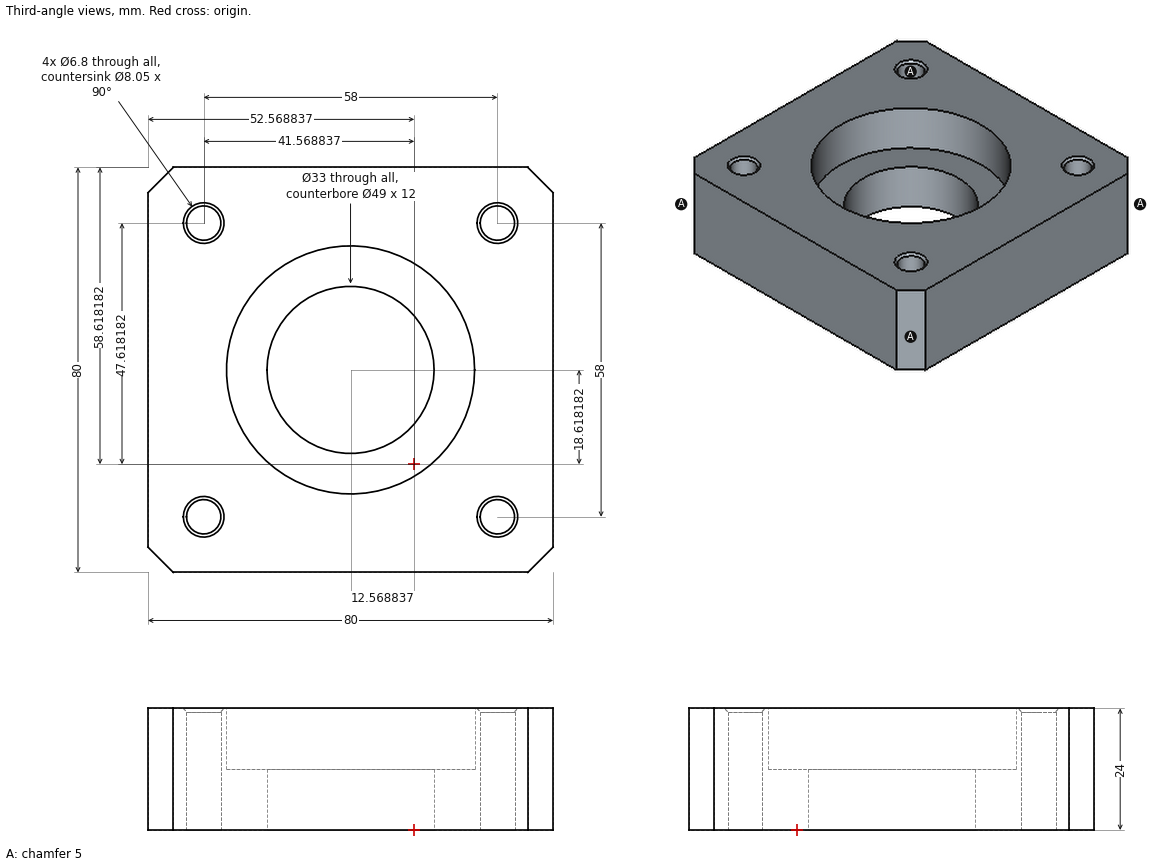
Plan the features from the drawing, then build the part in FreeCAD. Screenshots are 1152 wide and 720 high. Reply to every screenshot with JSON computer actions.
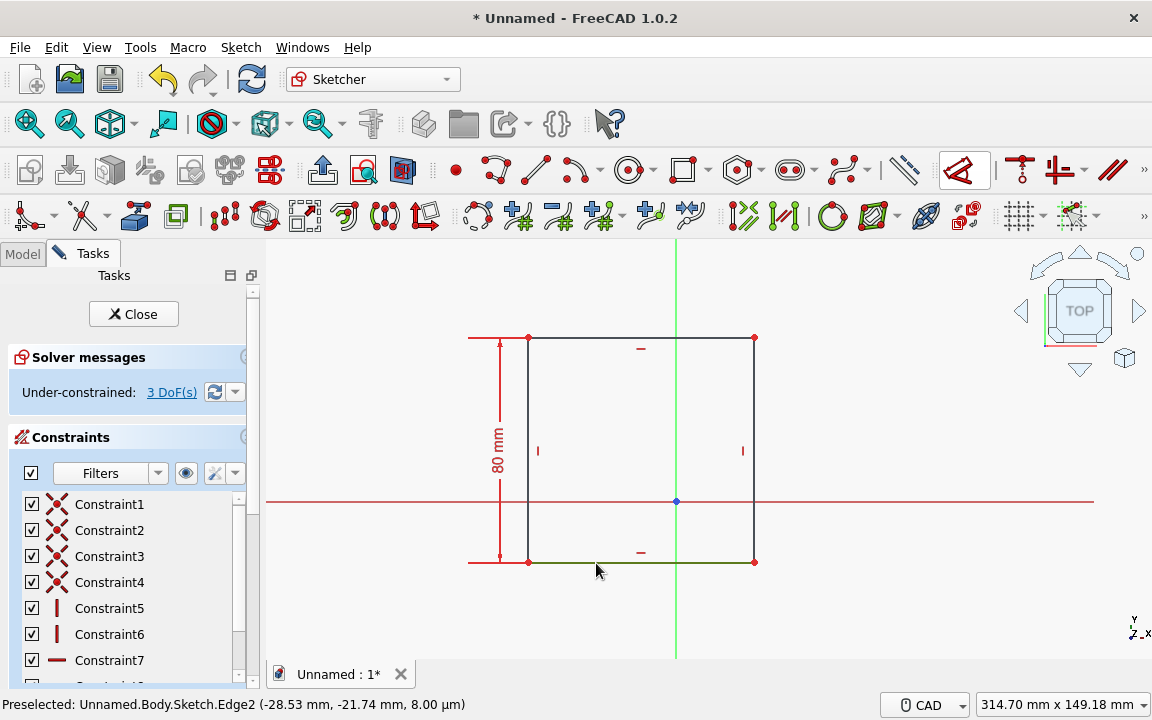
{"action": "key", "text": "l"}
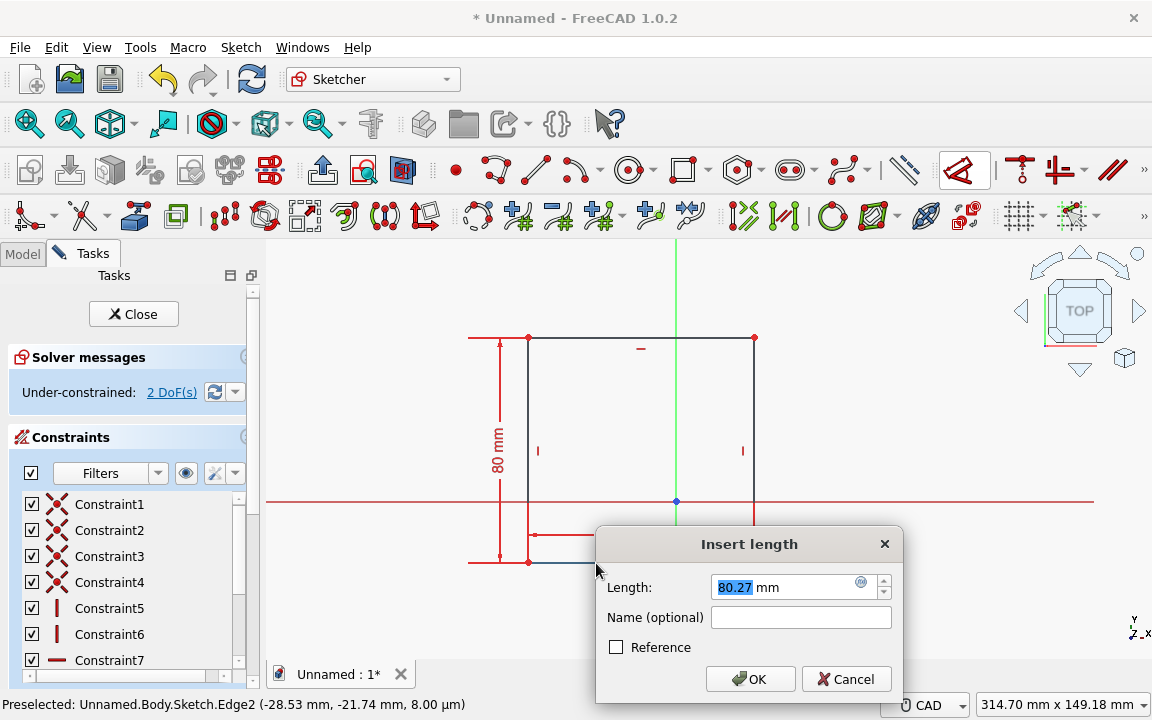
{"action": "type", "text": "80"}
{"action": "key", "text": "Return"}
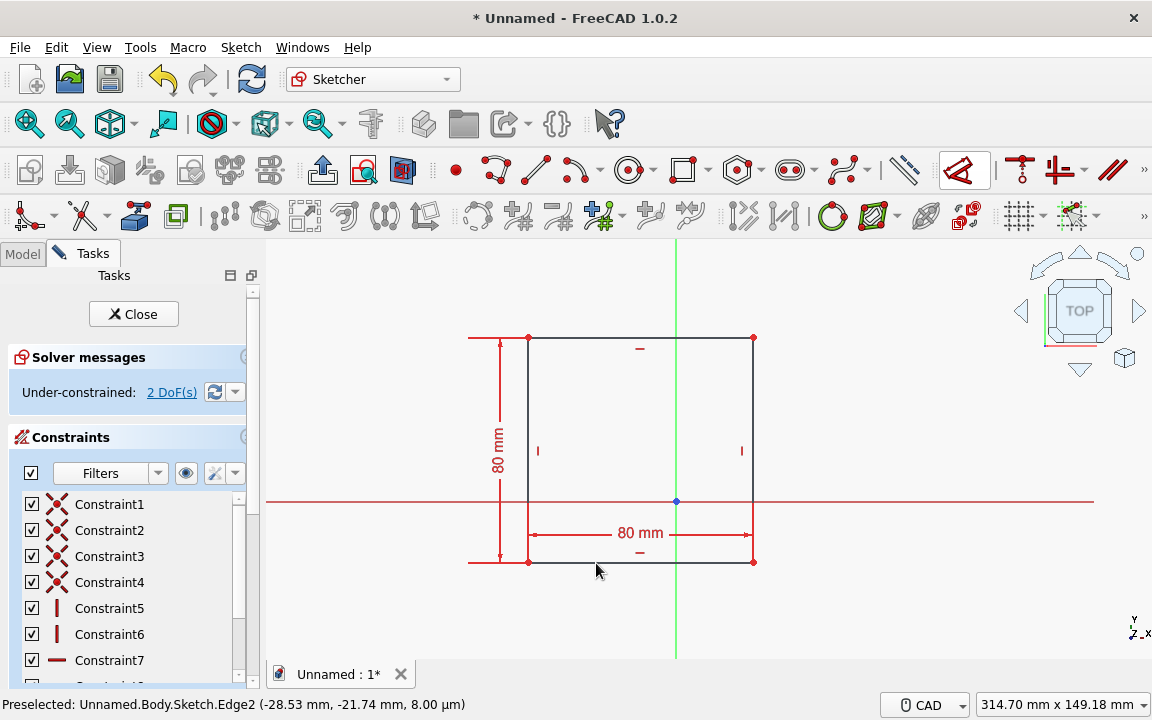
{"action": "left_click", "coordinate": [528, 338]}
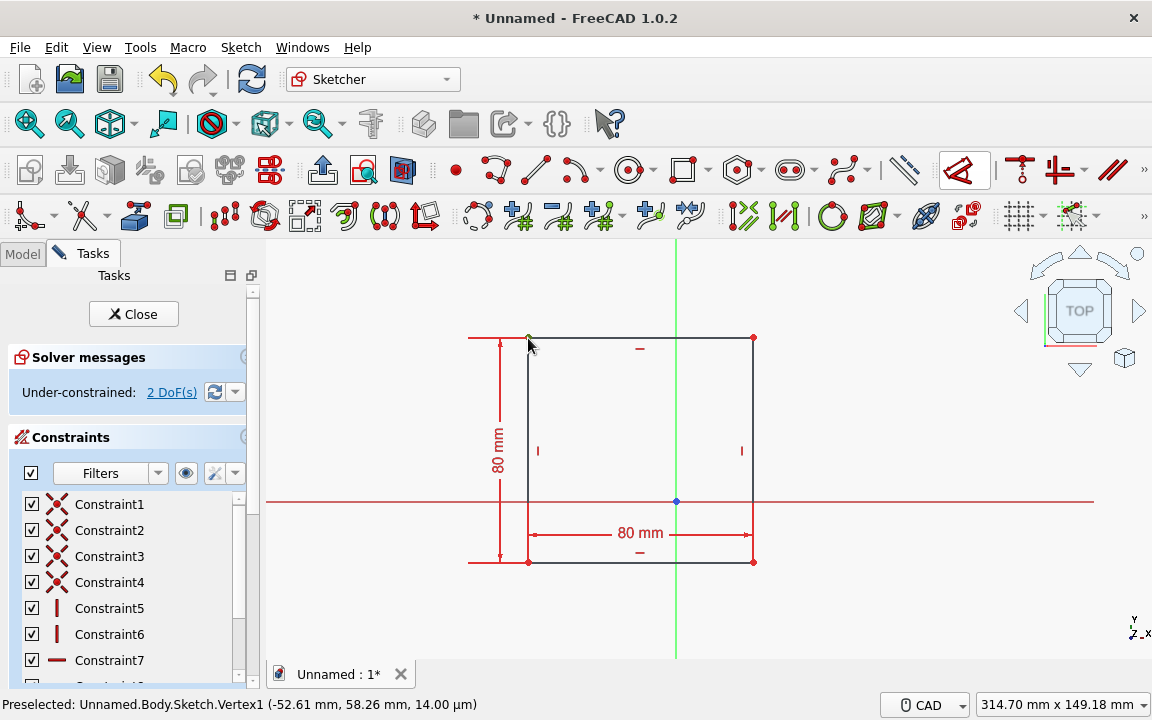
{"action": "left_click", "coordinate": [984, 170]}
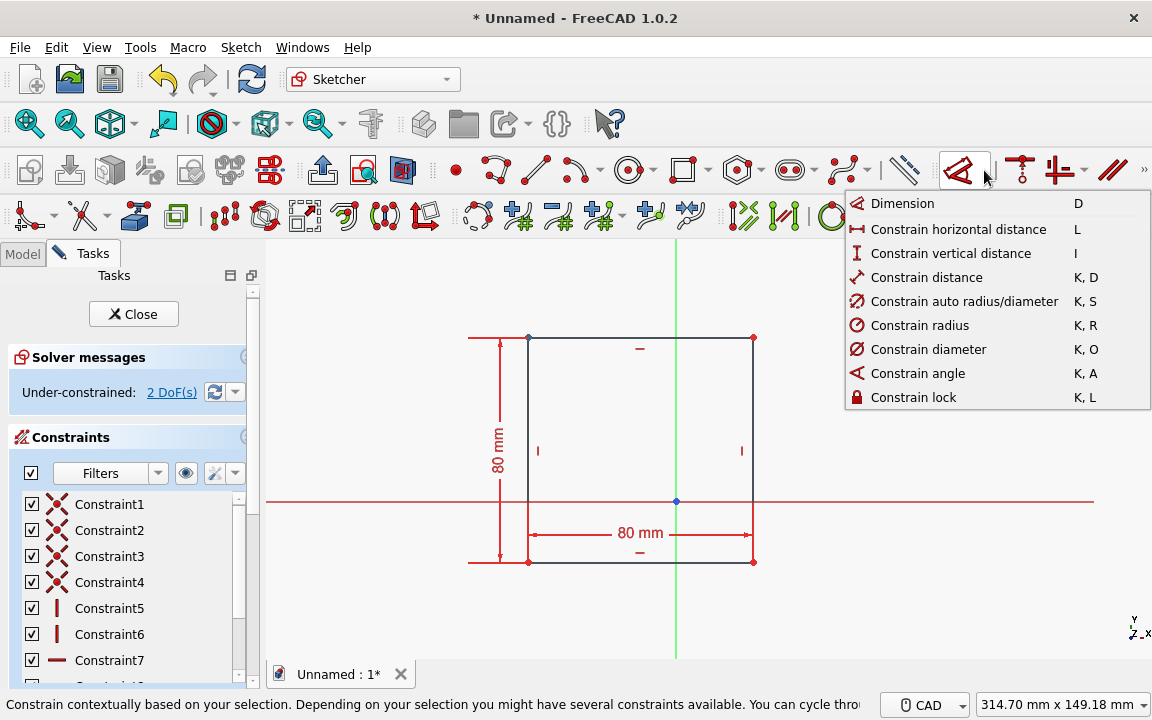
{"action": "left_click", "coordinate": [998, 229]}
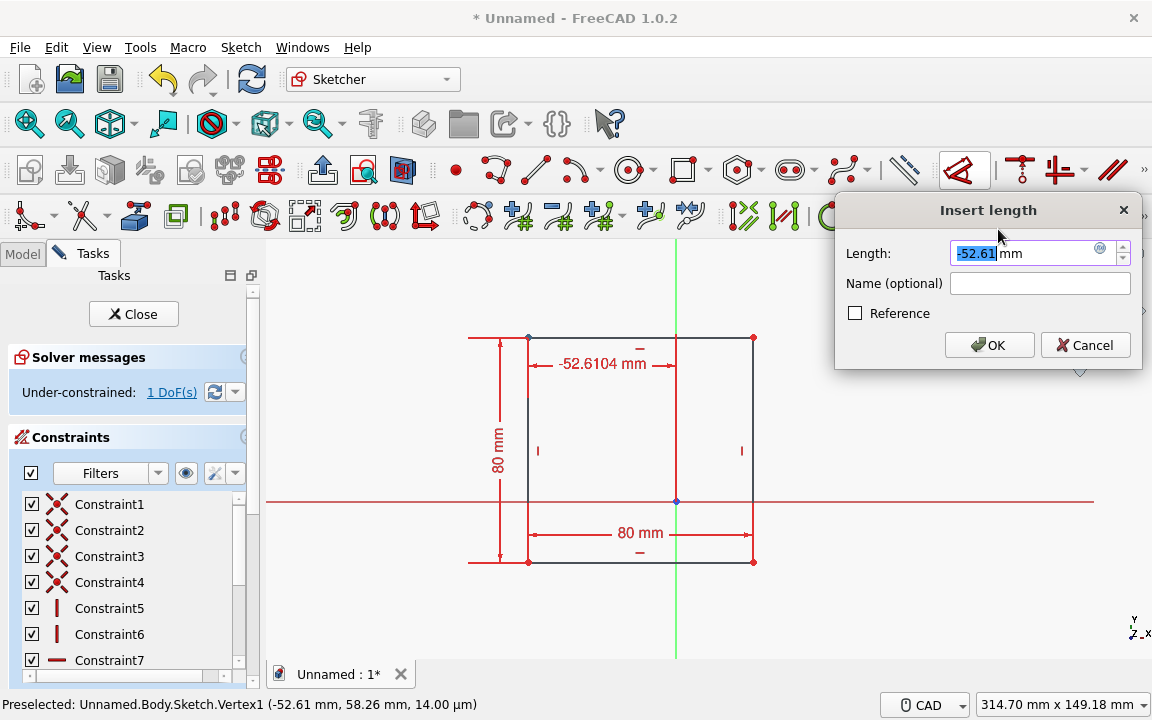
{"action": "type", "text": "-52.568837"}
{"action": "key", "text": "Return"}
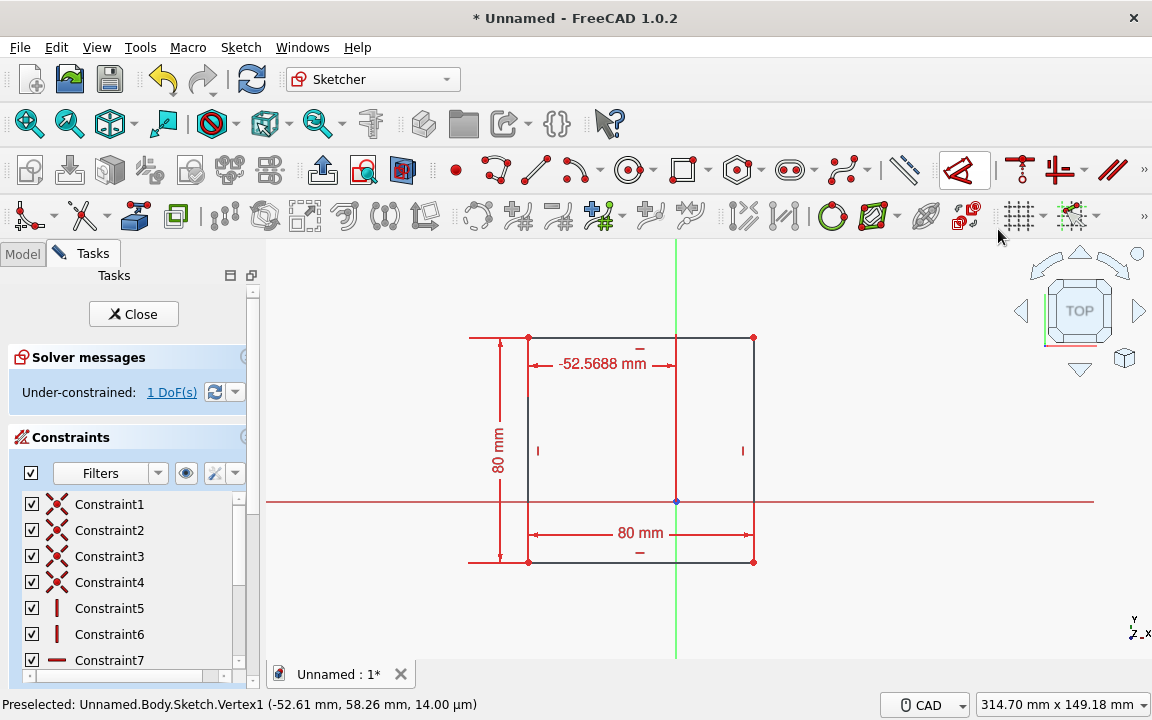
{"action": "left_click", "coordinate": [528, 338]}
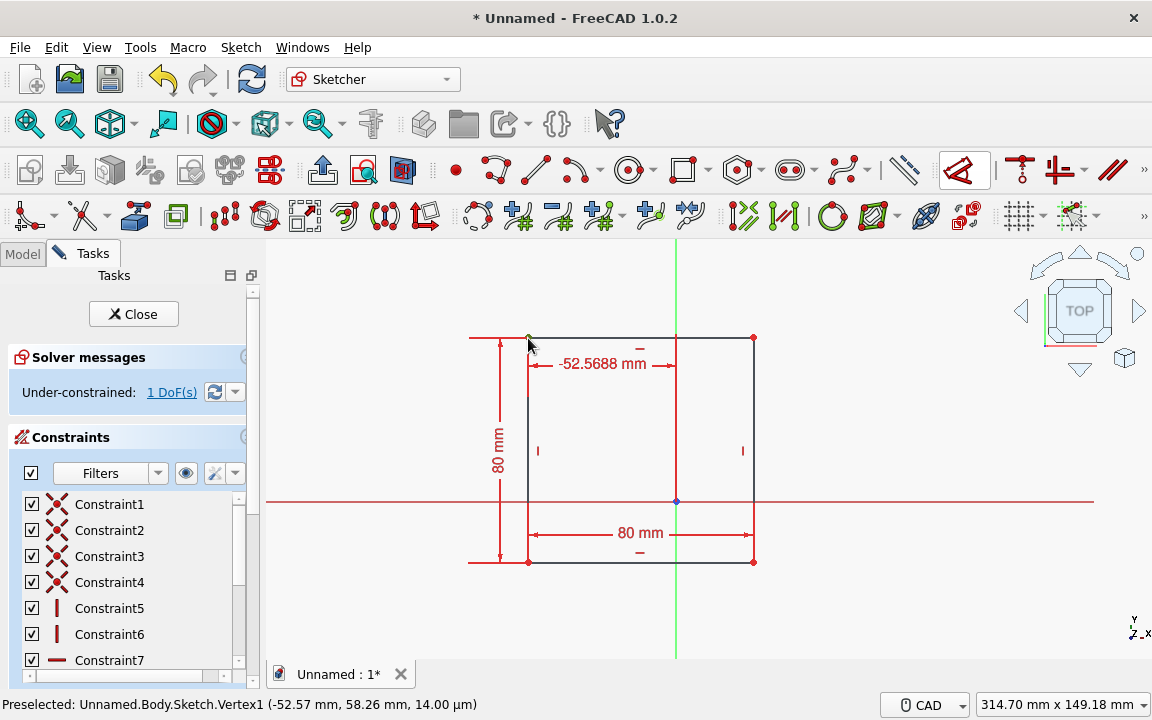
{"action": "key", "text": "i"}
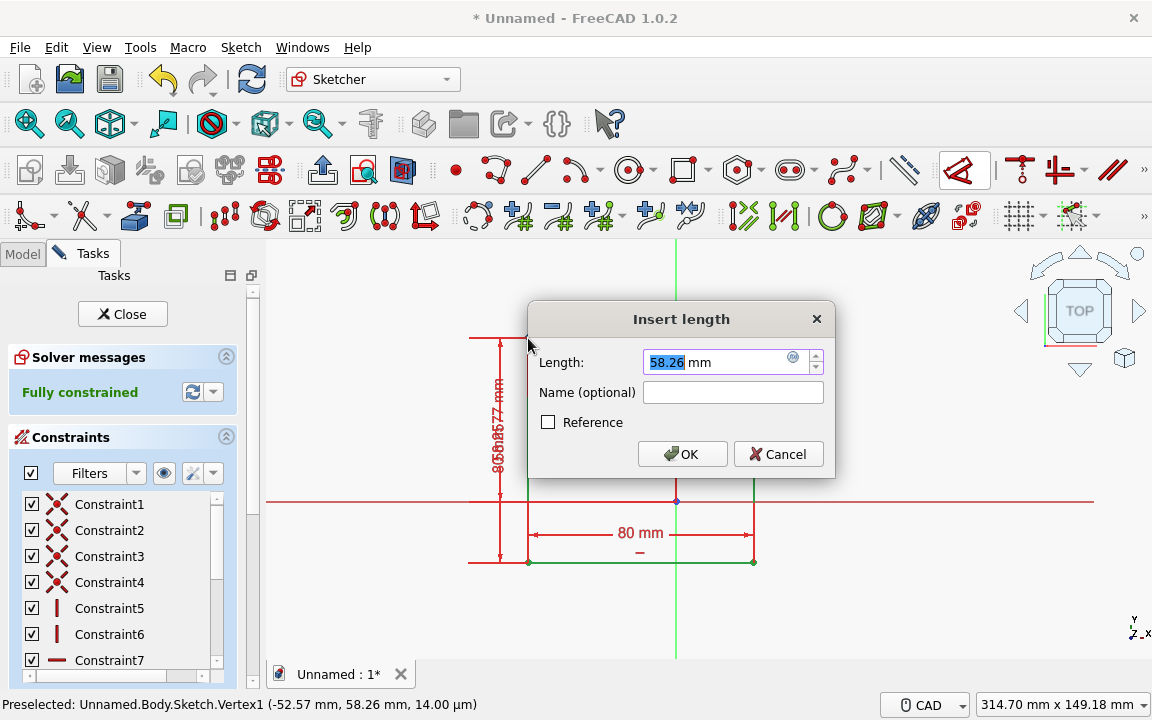
{"action": "type", "text": "58.618182"}
{"action": "key", "text": "Return"}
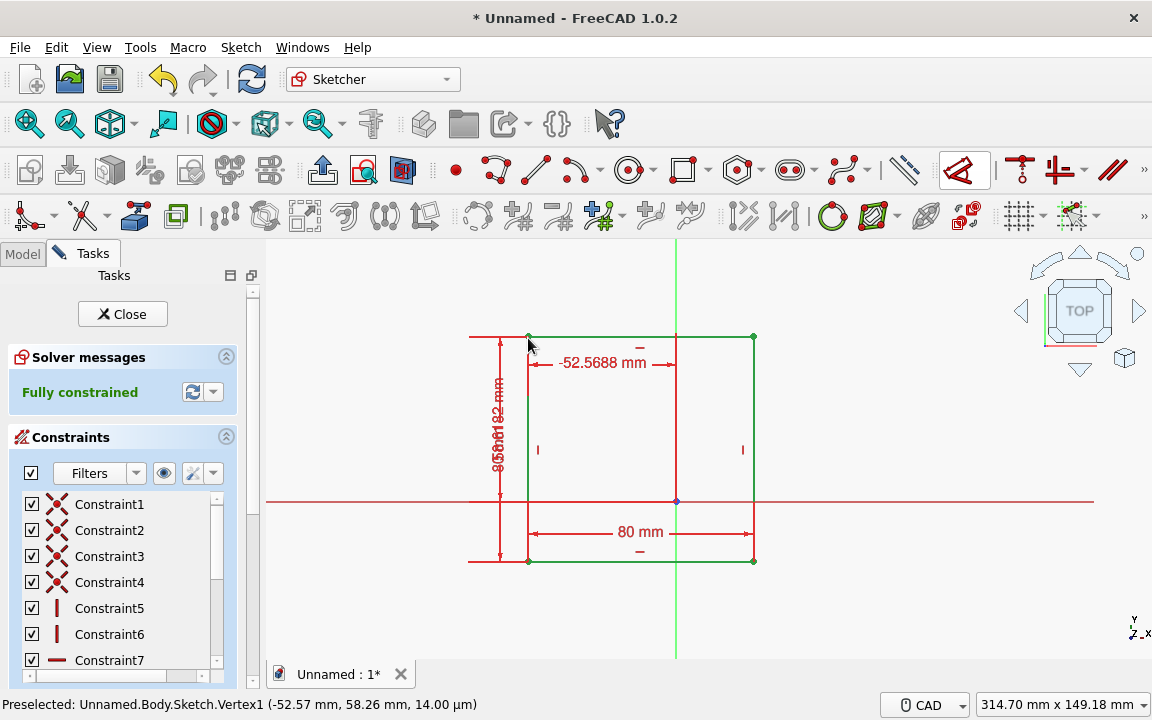
{"action": "left_click", "coordinate": [123, 314]}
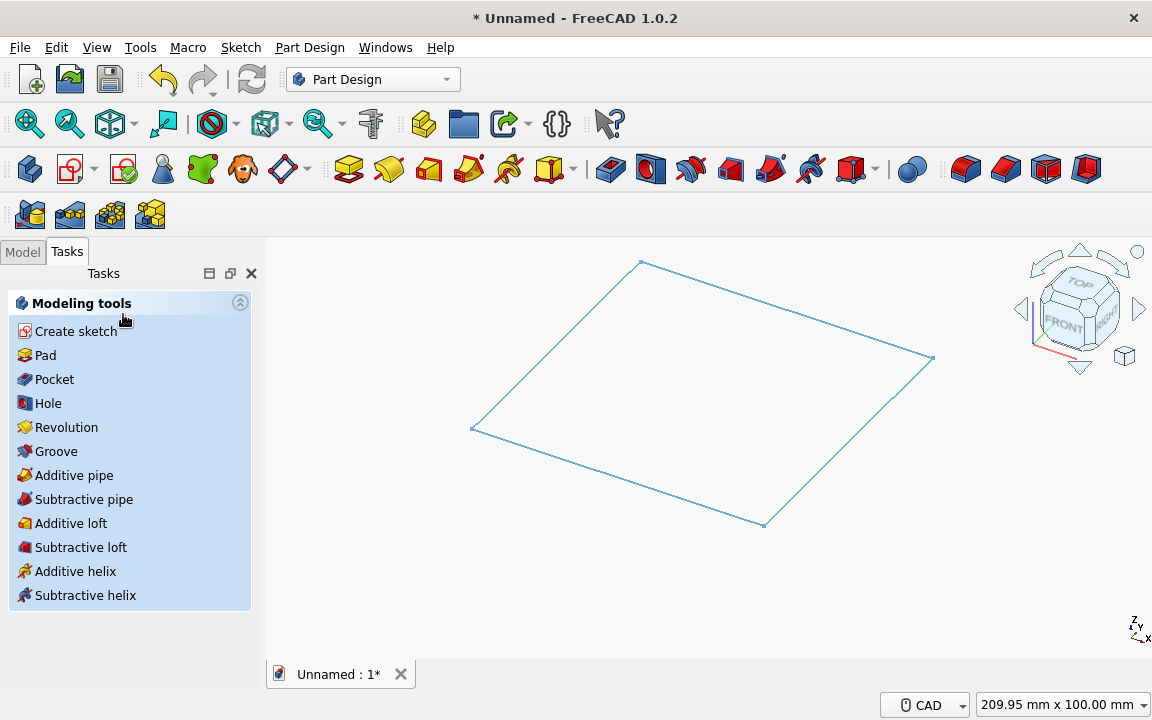
{"action": "left_click", "coordinate": [350, 170]}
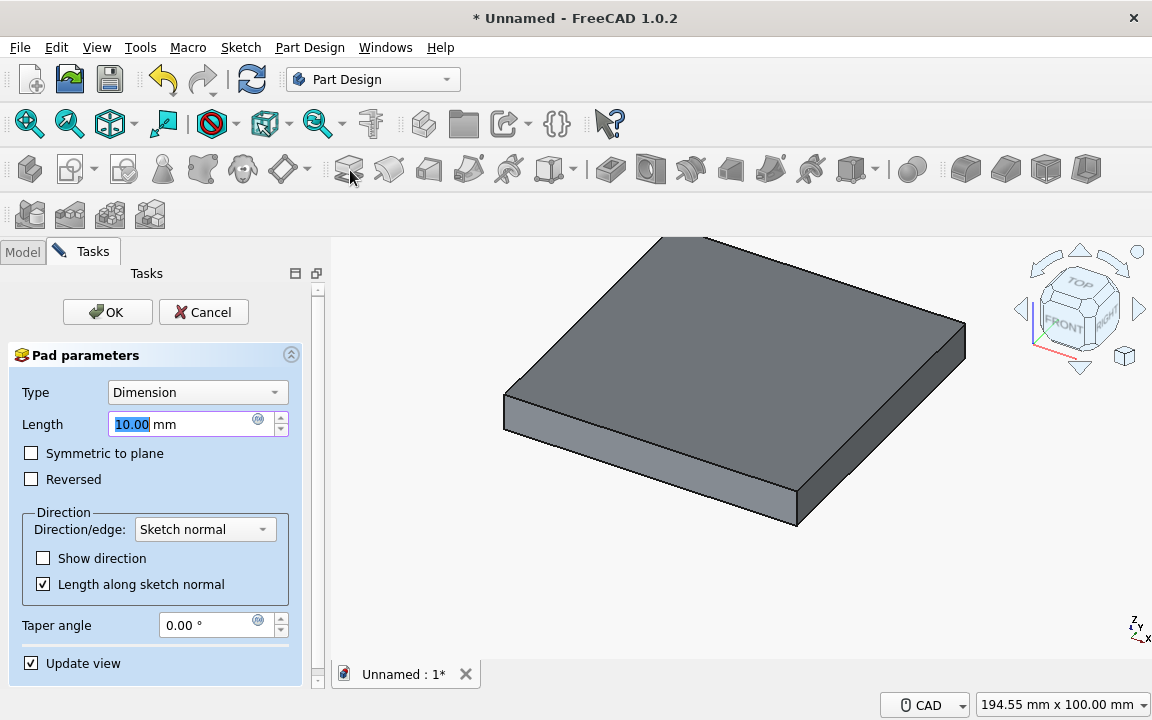
{"action": "type", "text": "24"}
{"action": "key", "text": "Tab"}